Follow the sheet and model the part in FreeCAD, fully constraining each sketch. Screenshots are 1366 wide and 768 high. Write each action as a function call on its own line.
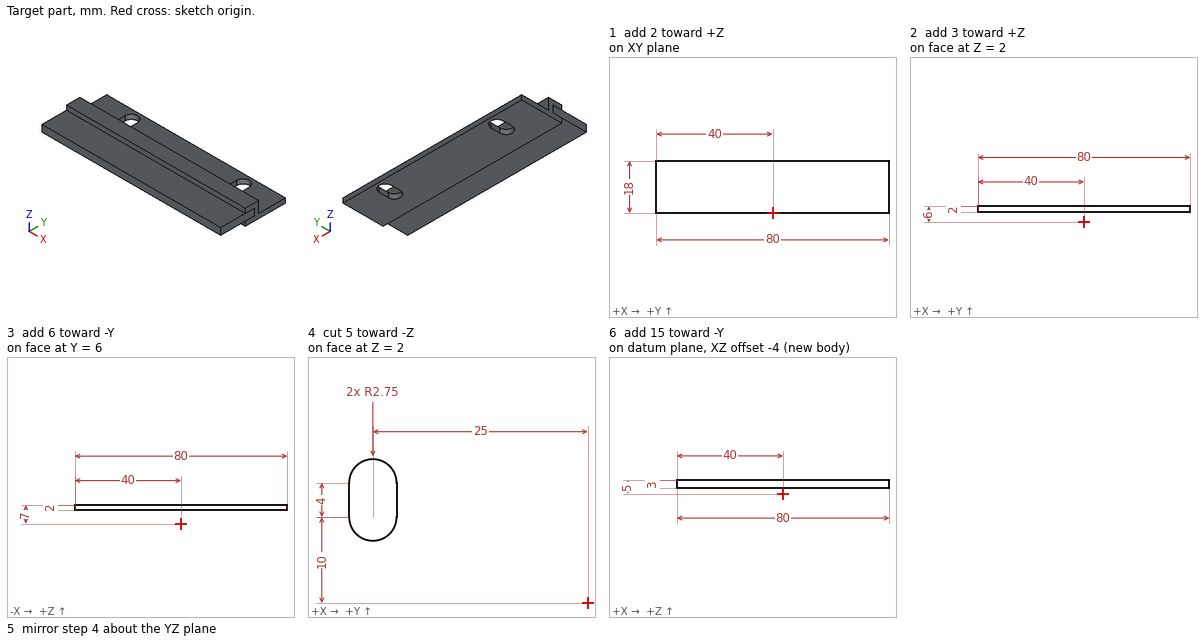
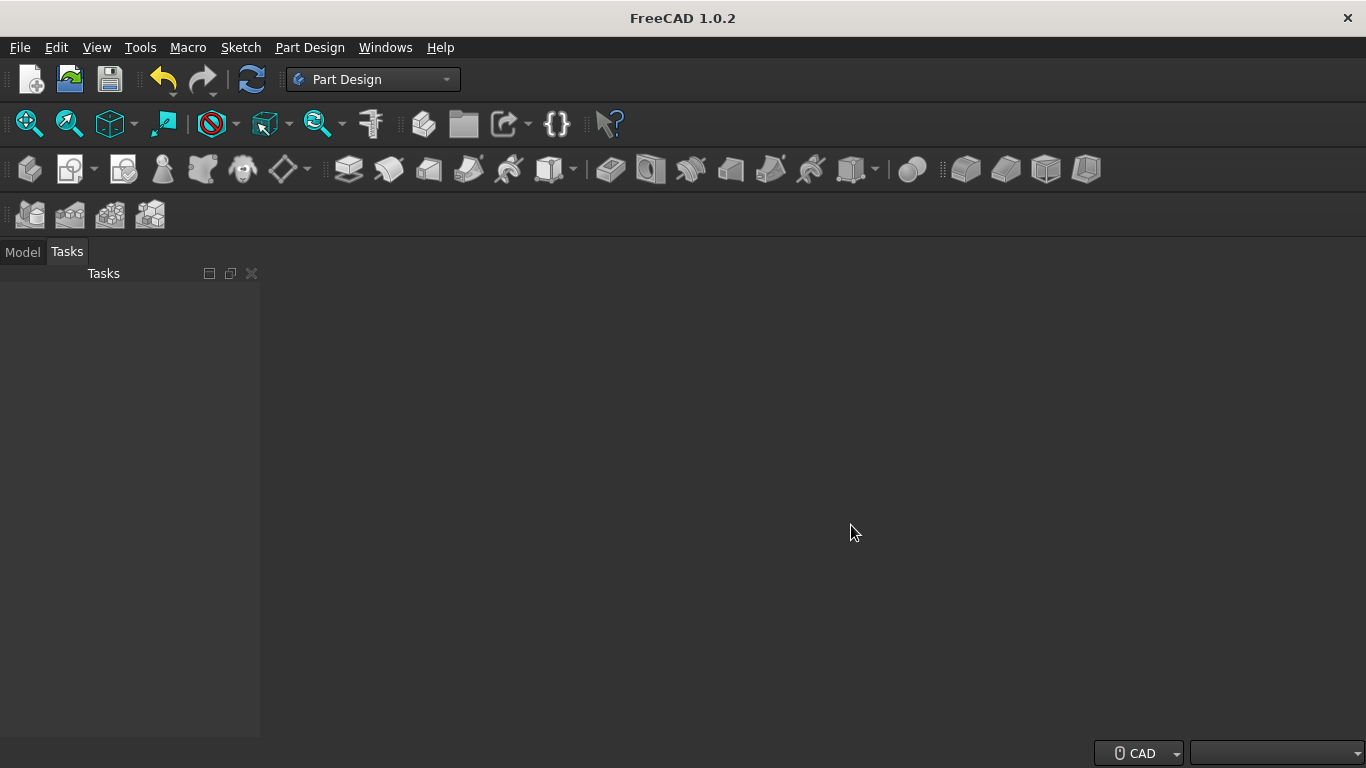
key(ctrl+n)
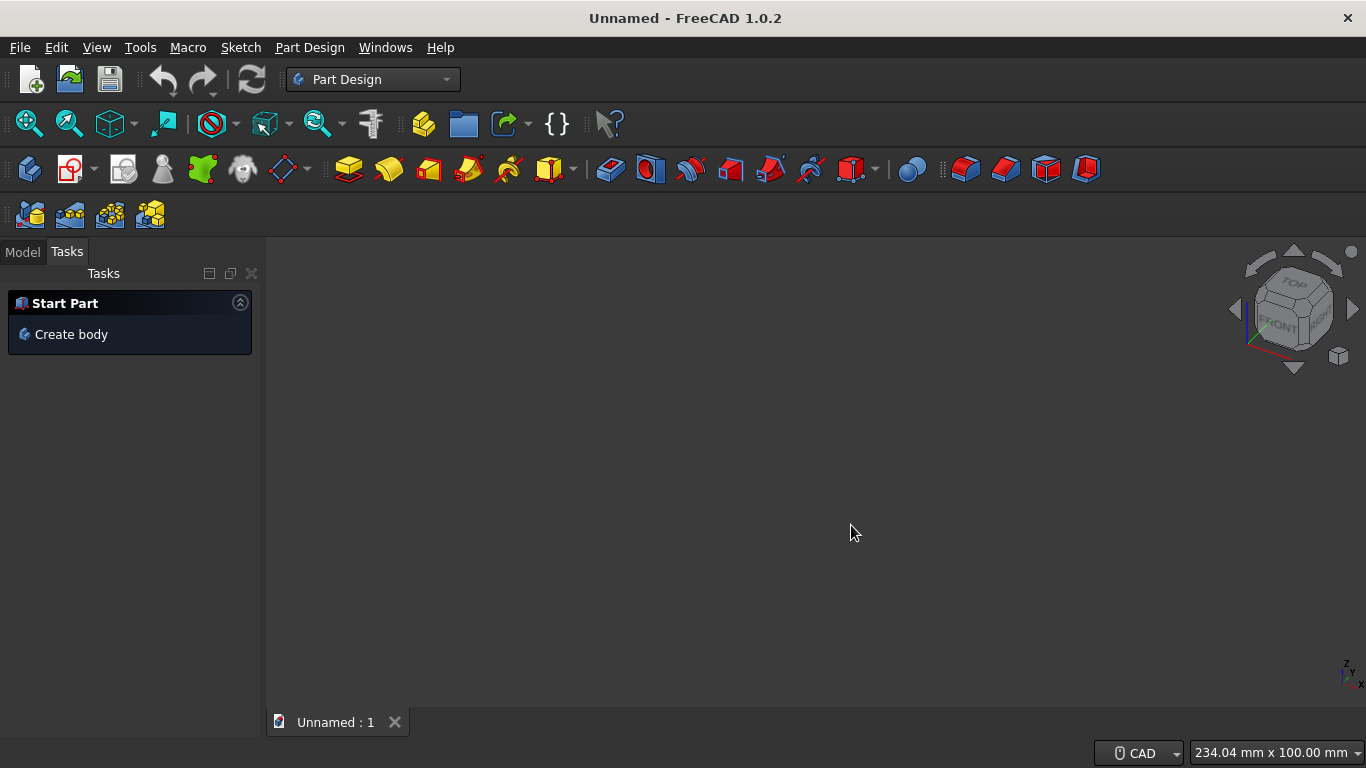
click(70, 170)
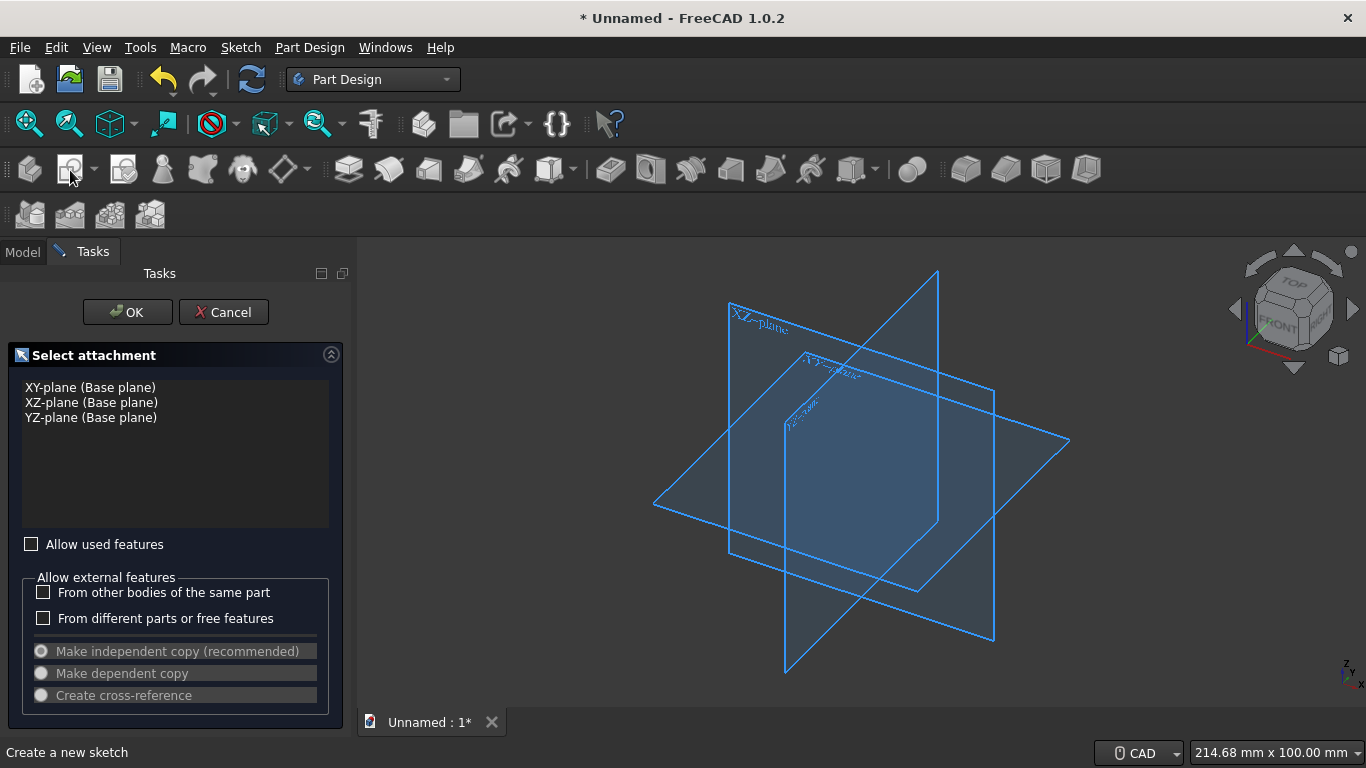
click(82, 388)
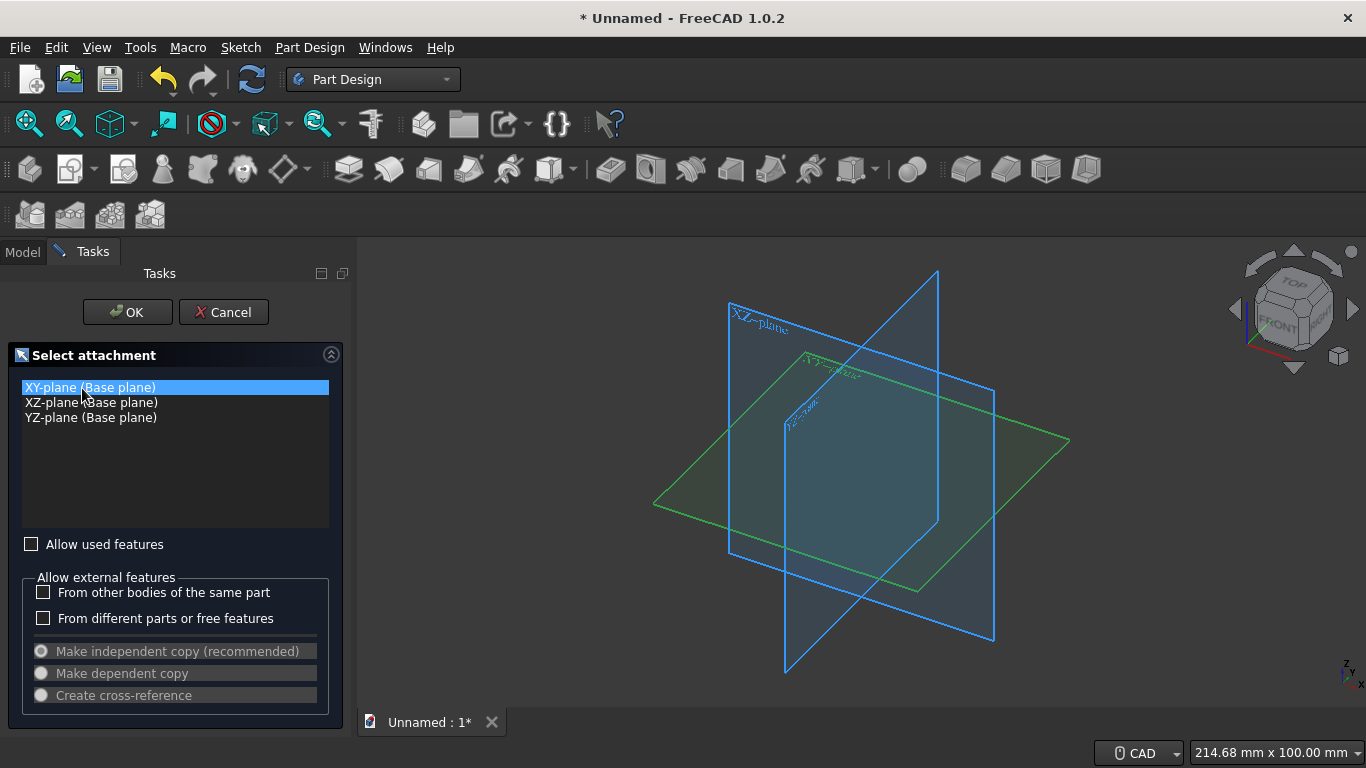
click(128, 312)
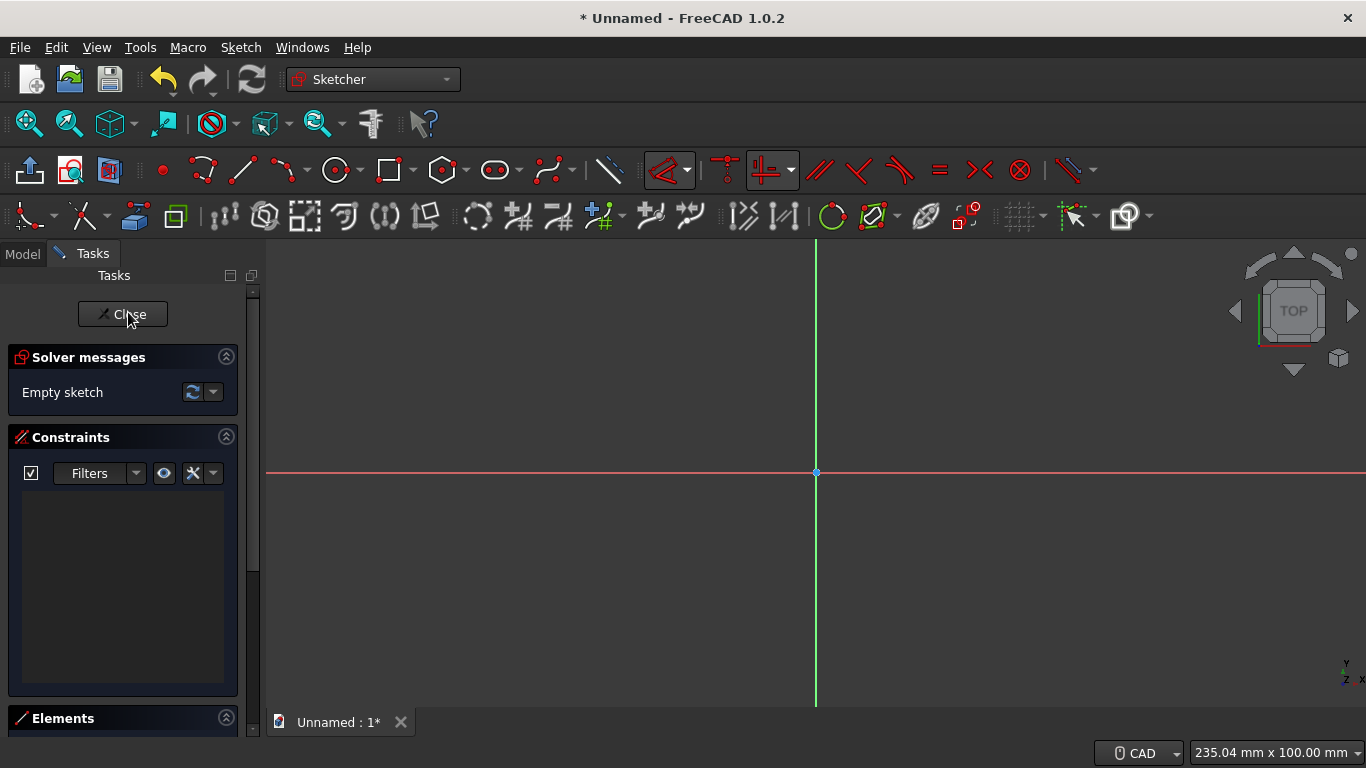
scroll(899, 380, up, 3)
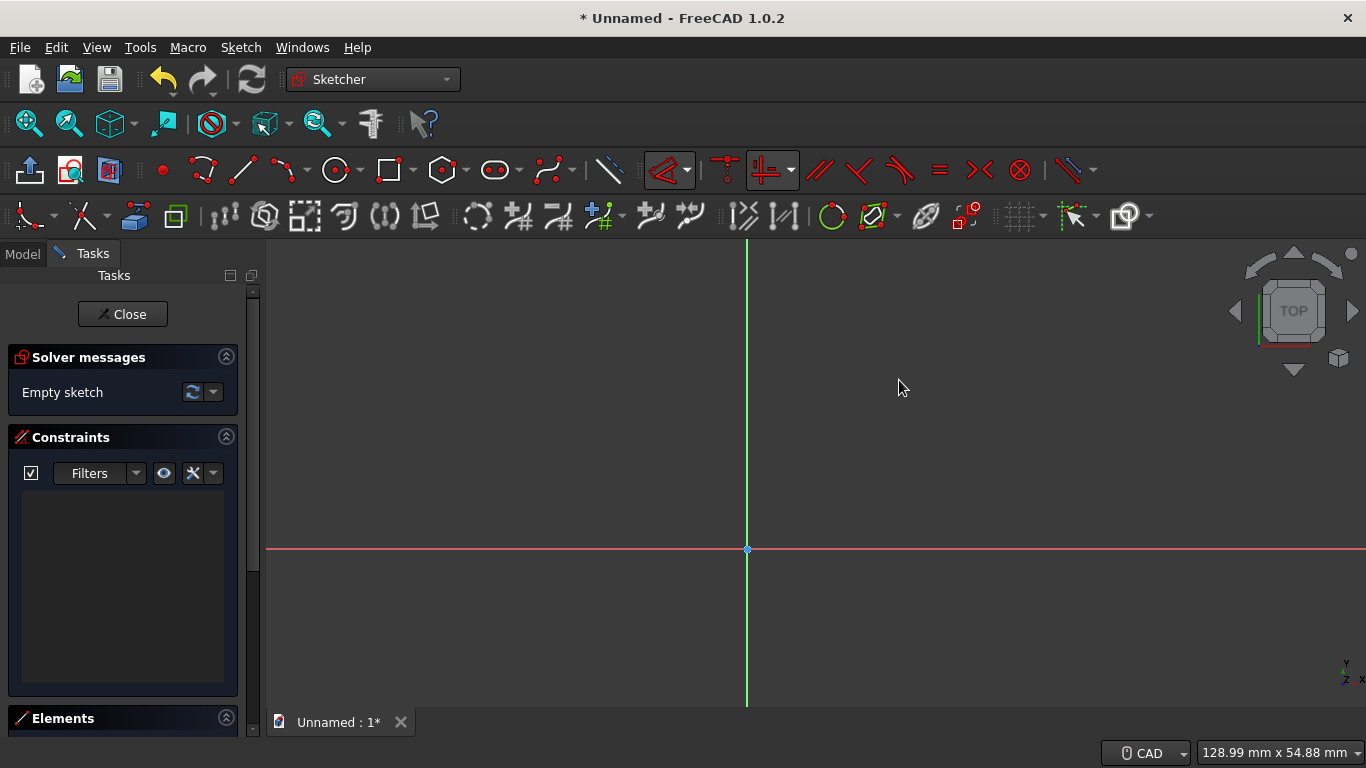
click(390, 170)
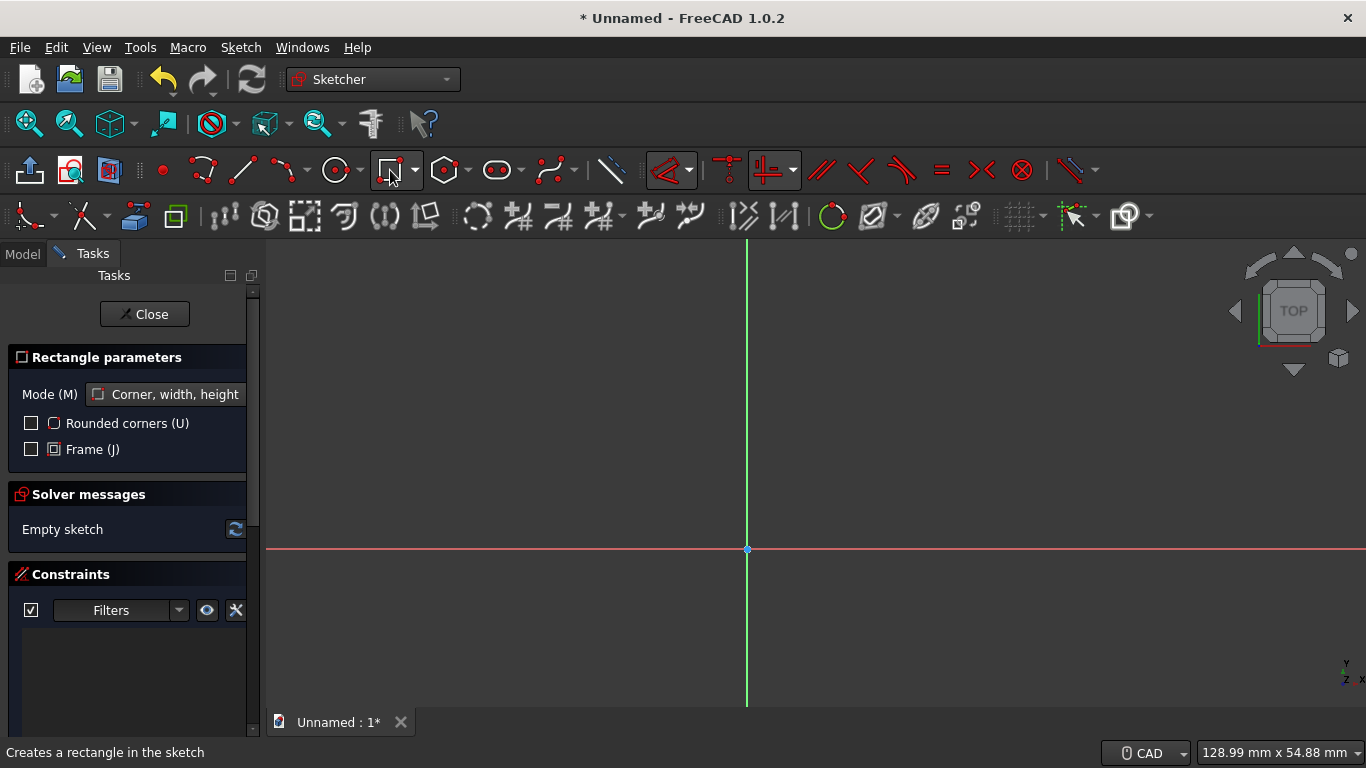
click(406, 396)
click(1088, 549)
key(Escape)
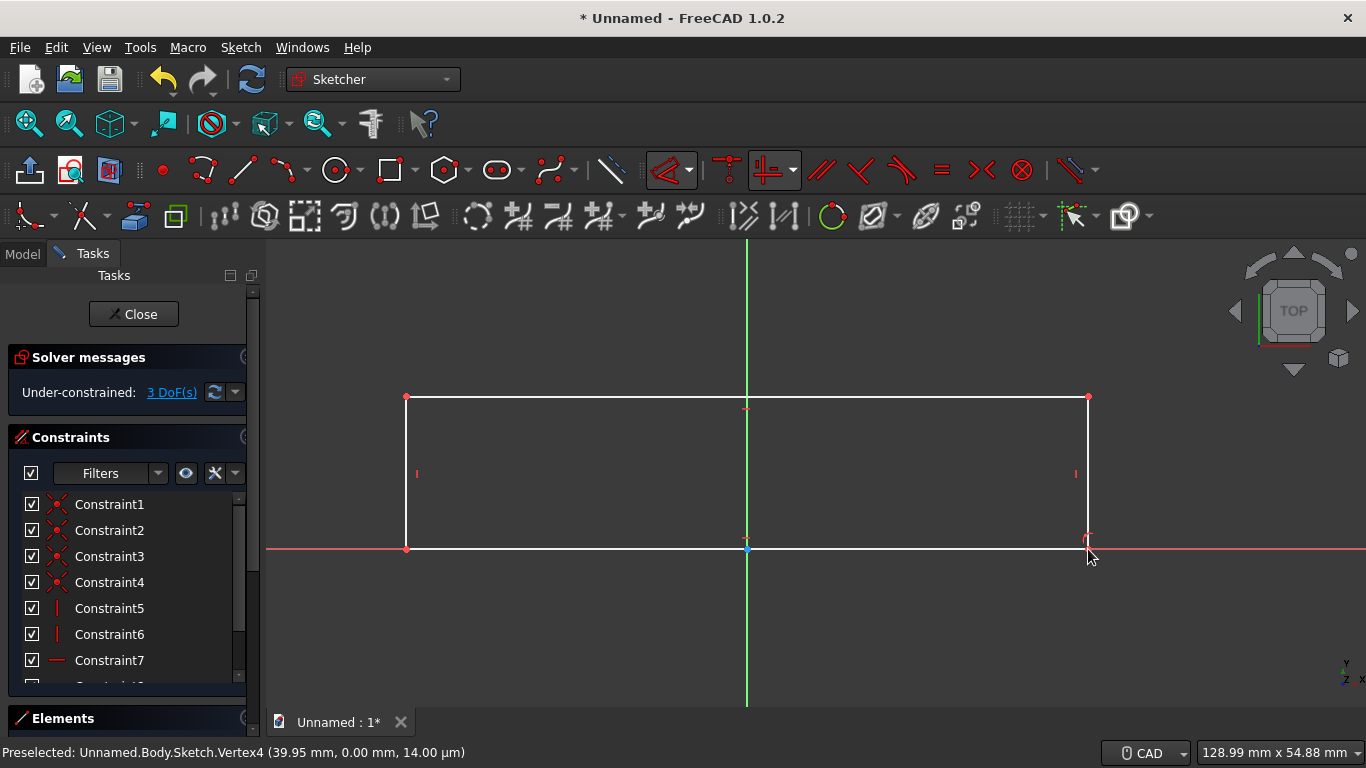
click(406, 443)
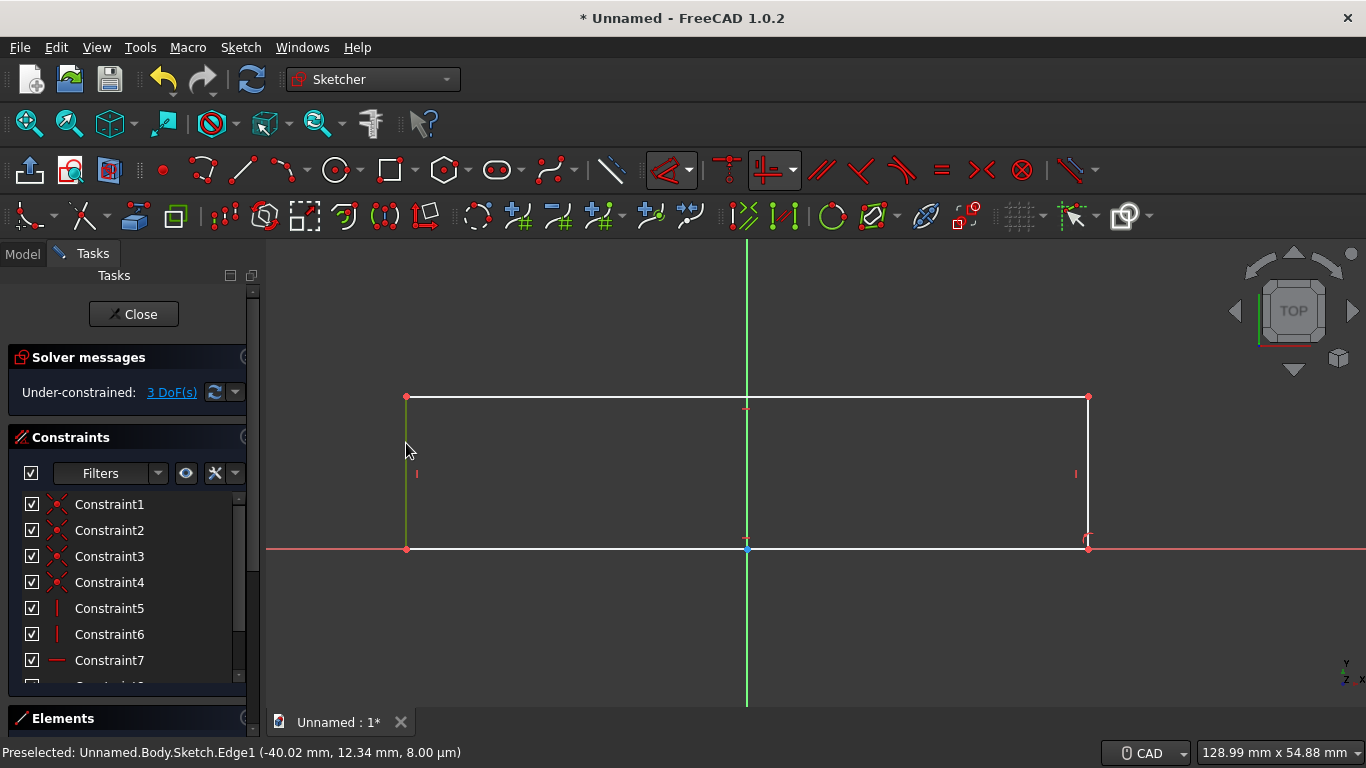
click(692, 170)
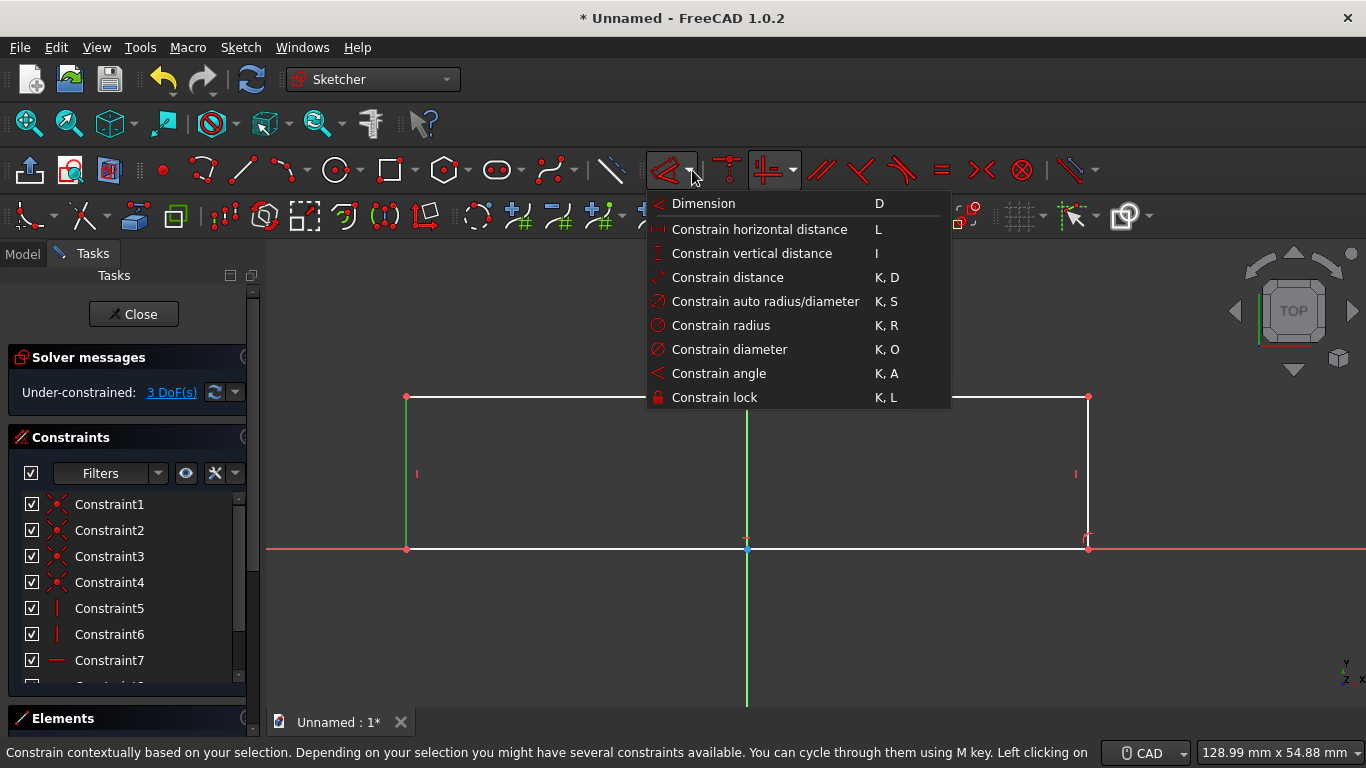
click(799, 253)